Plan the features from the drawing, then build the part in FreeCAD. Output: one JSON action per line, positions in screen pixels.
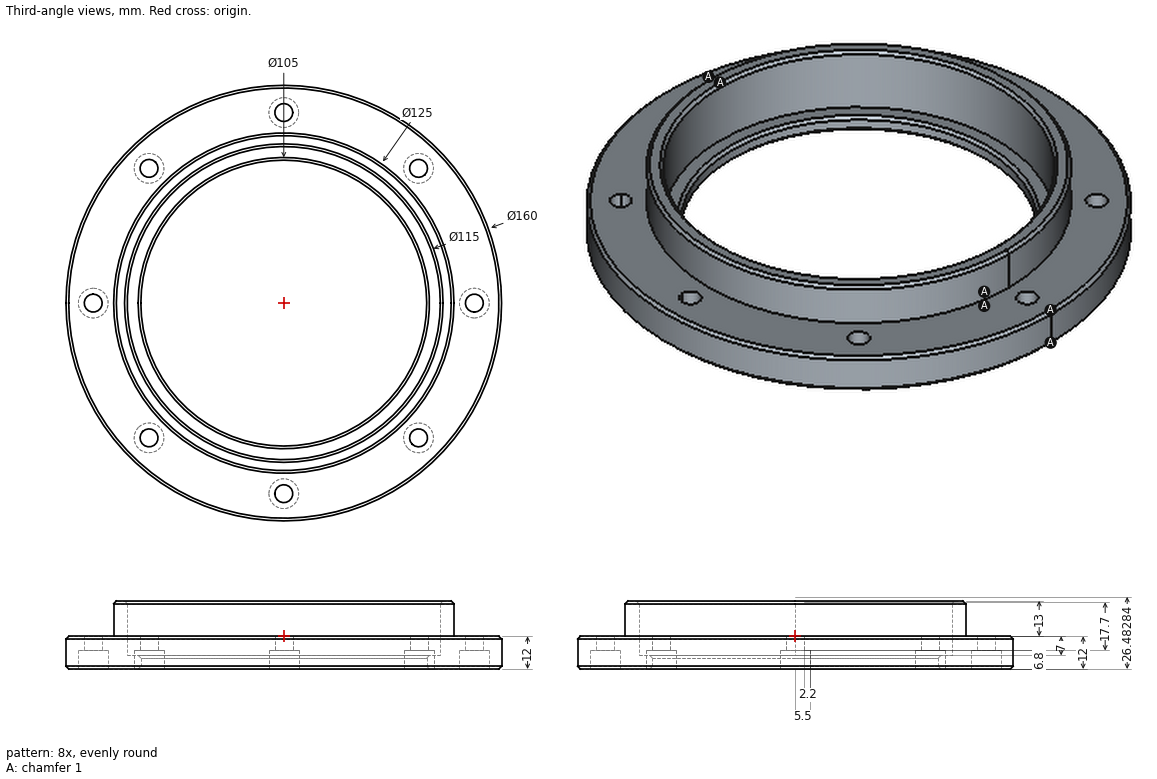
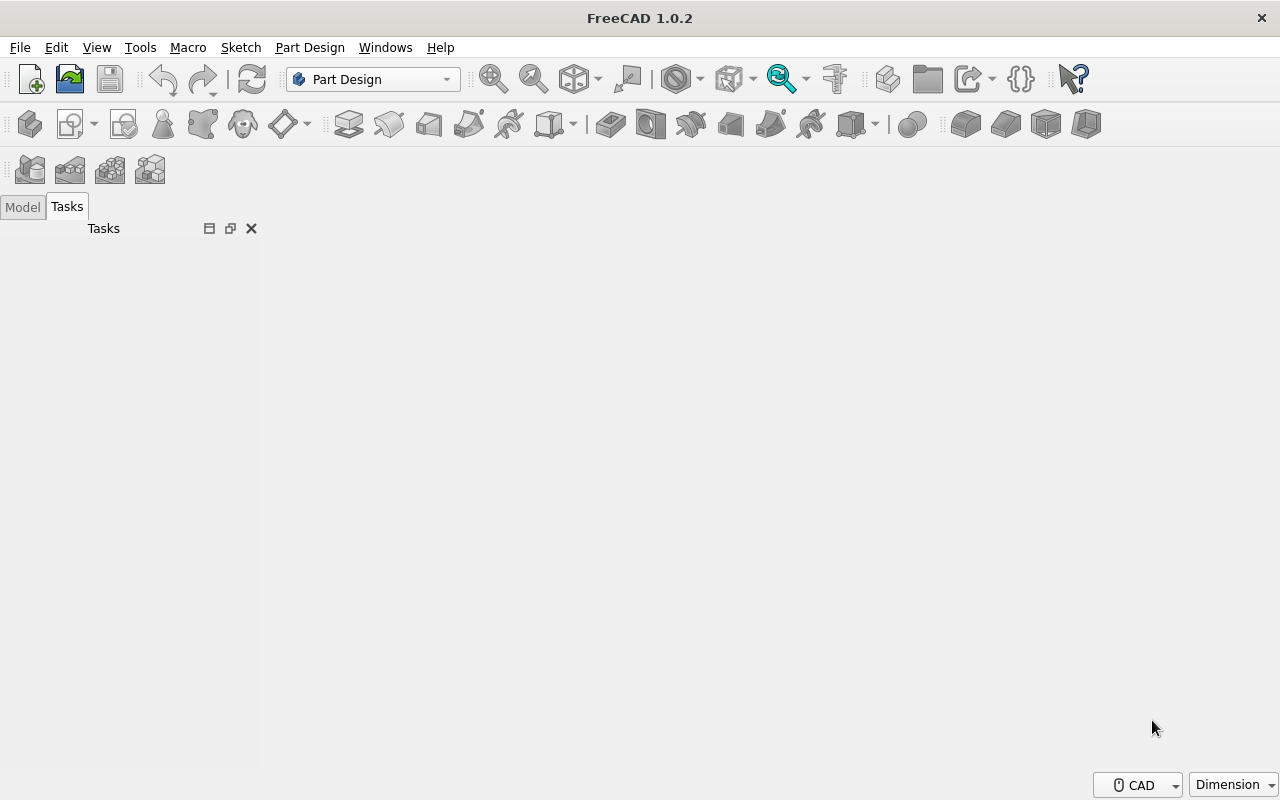
{"action": "key", "text": "ctrl+n"}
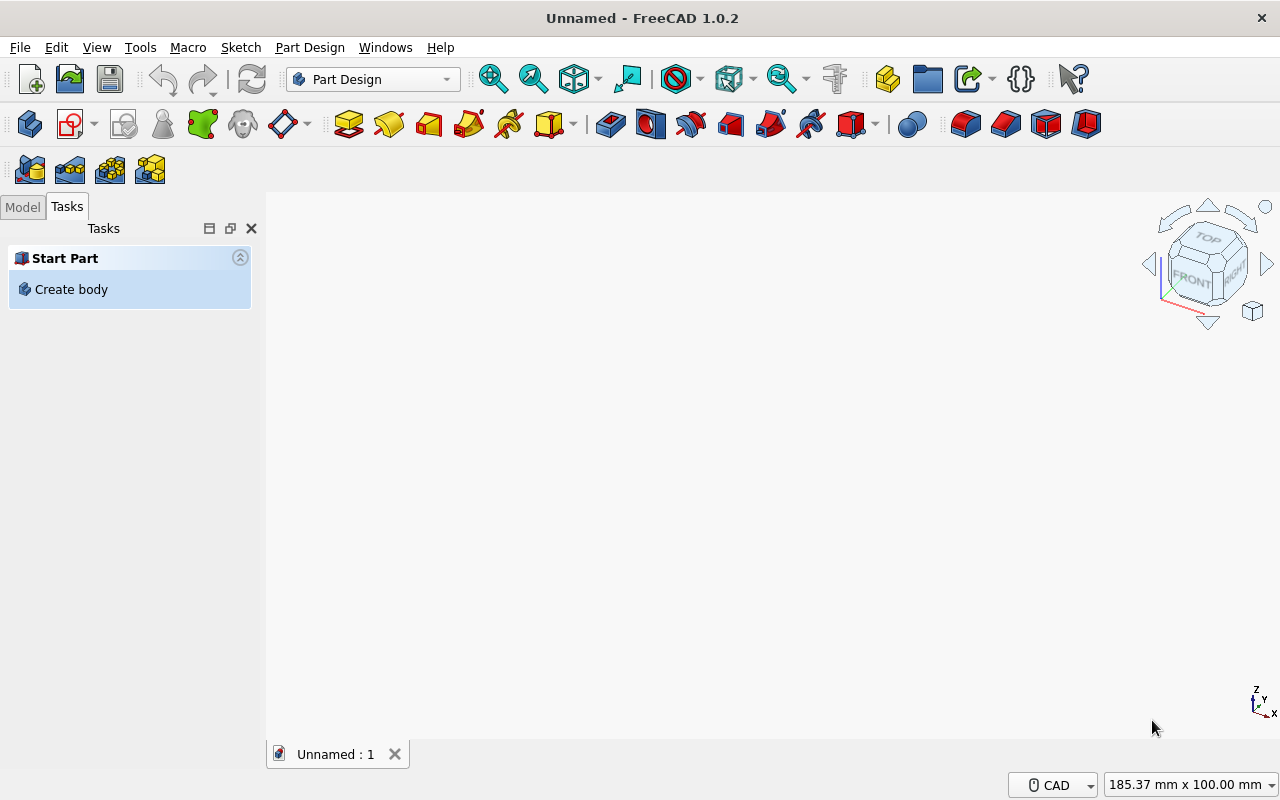
{"action": "left_click", "coordinate": [70, 124]}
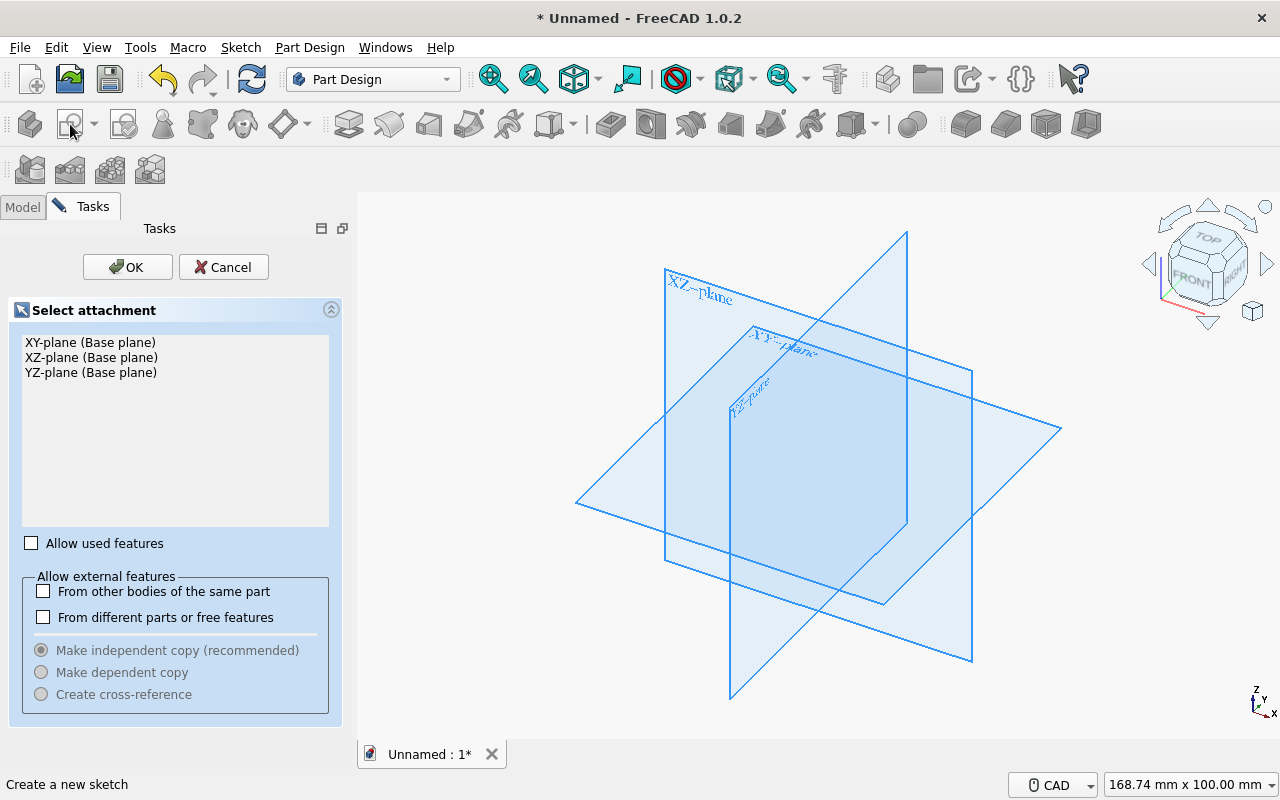
{"action": "left_click", "coordinate": [82, 342]}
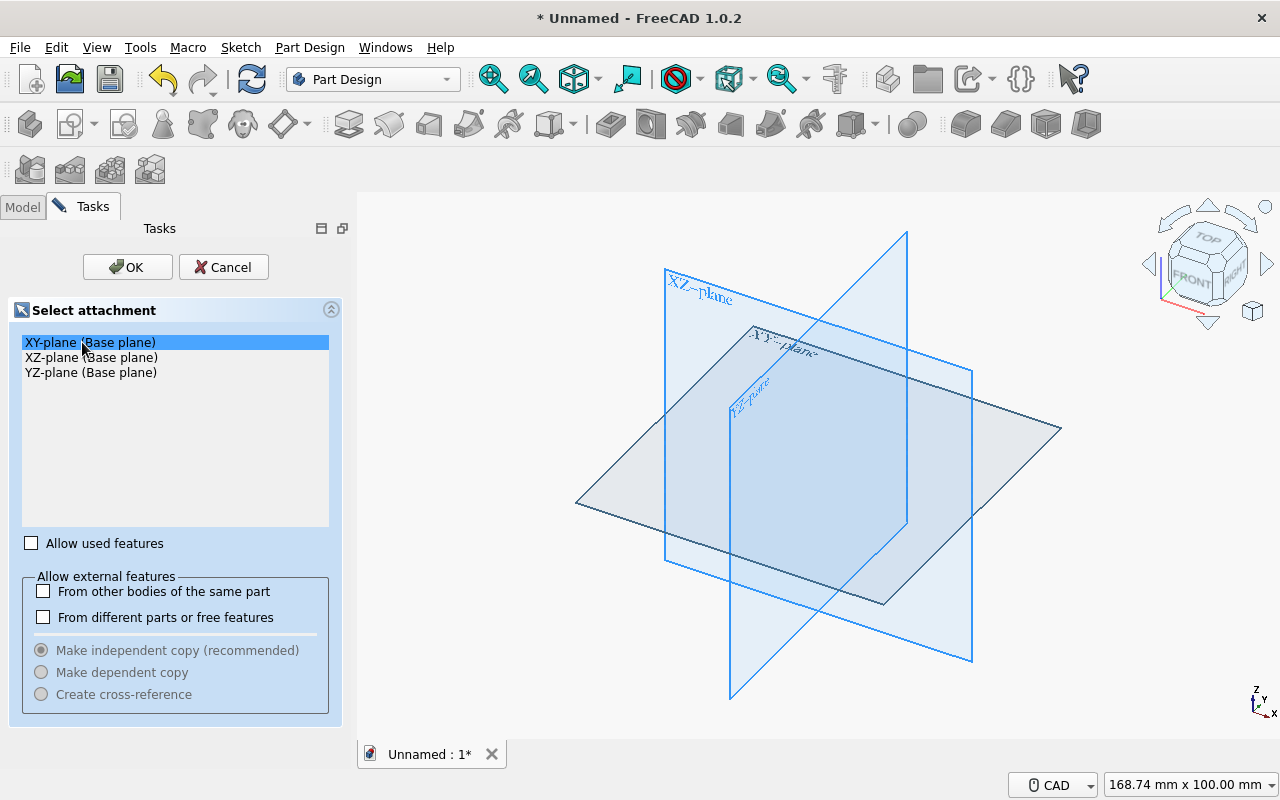
{"action": "left_click", "coordinate": [128, 267]}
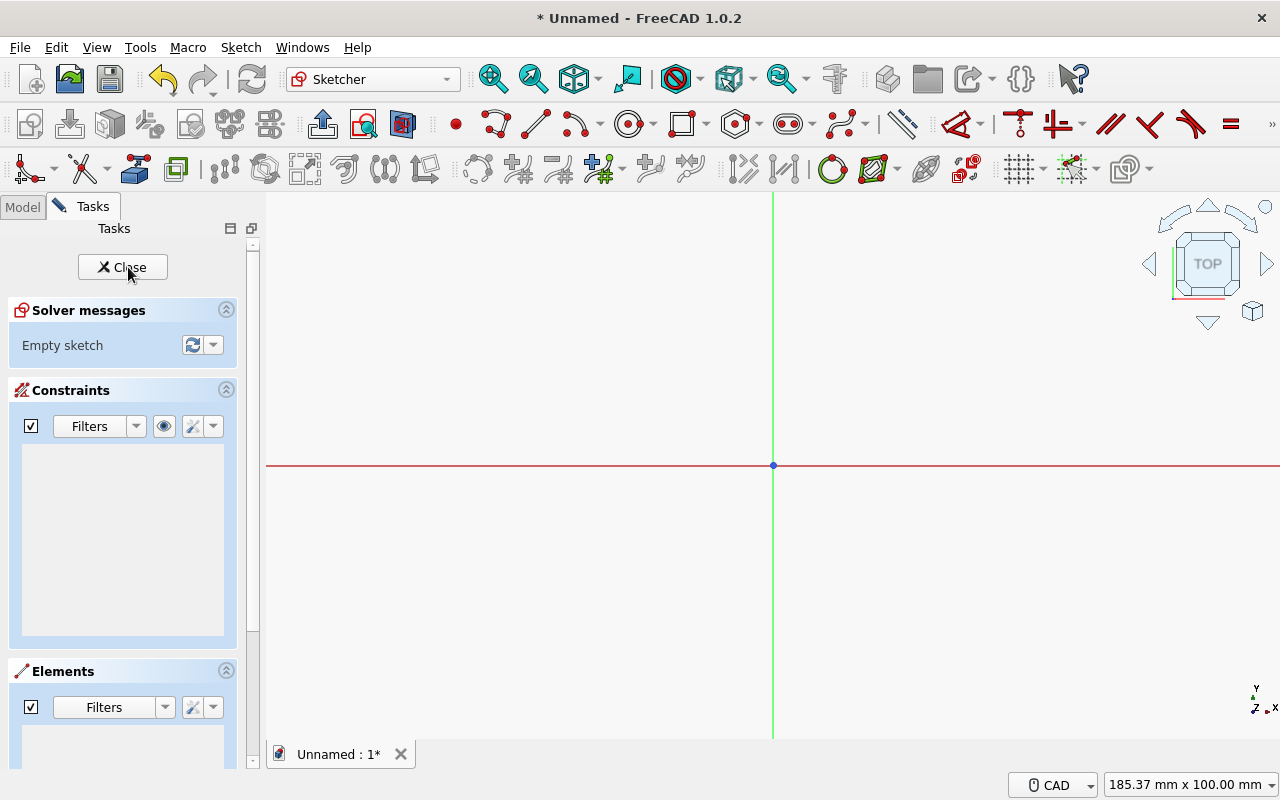
{"action": "scroll", "coordinate": [621, 466], "scroll_direction": "down", "scroll_amount": 3}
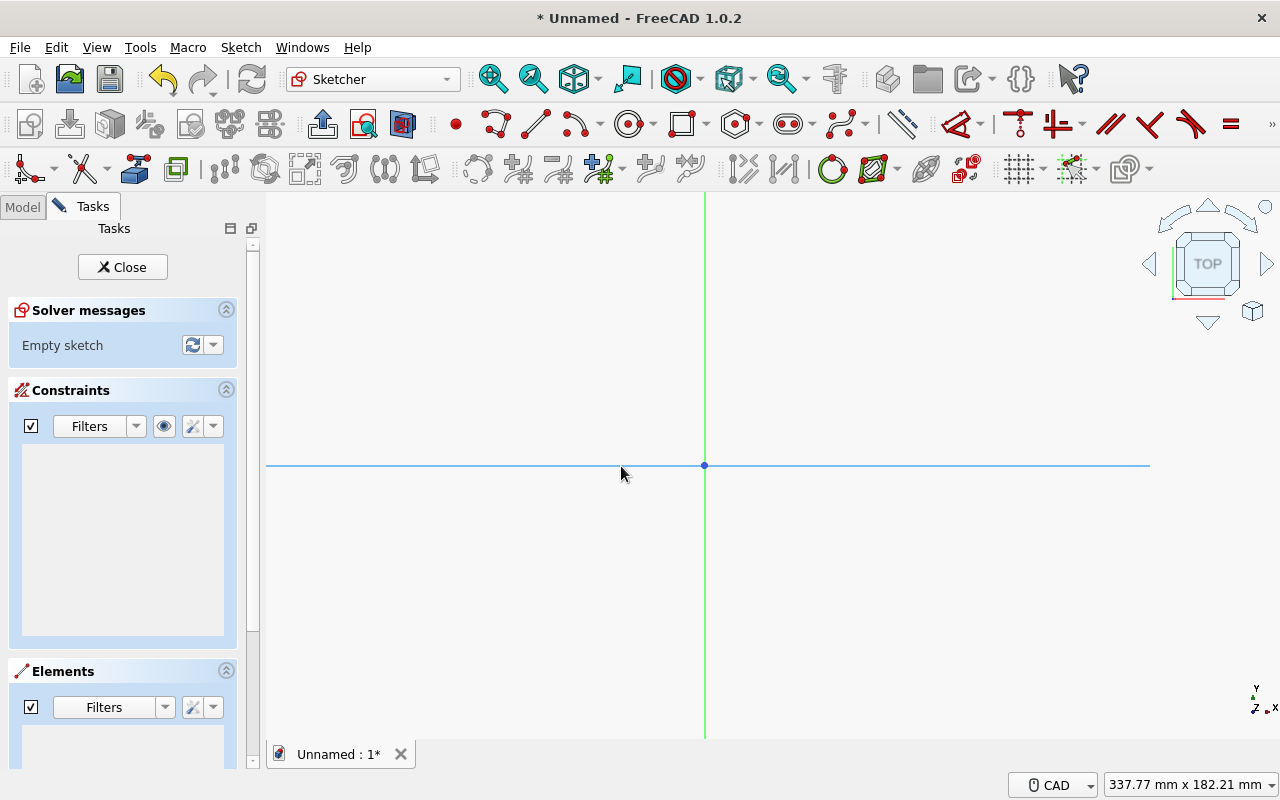
{"action": "left_click", "coordinate": [630, 124]}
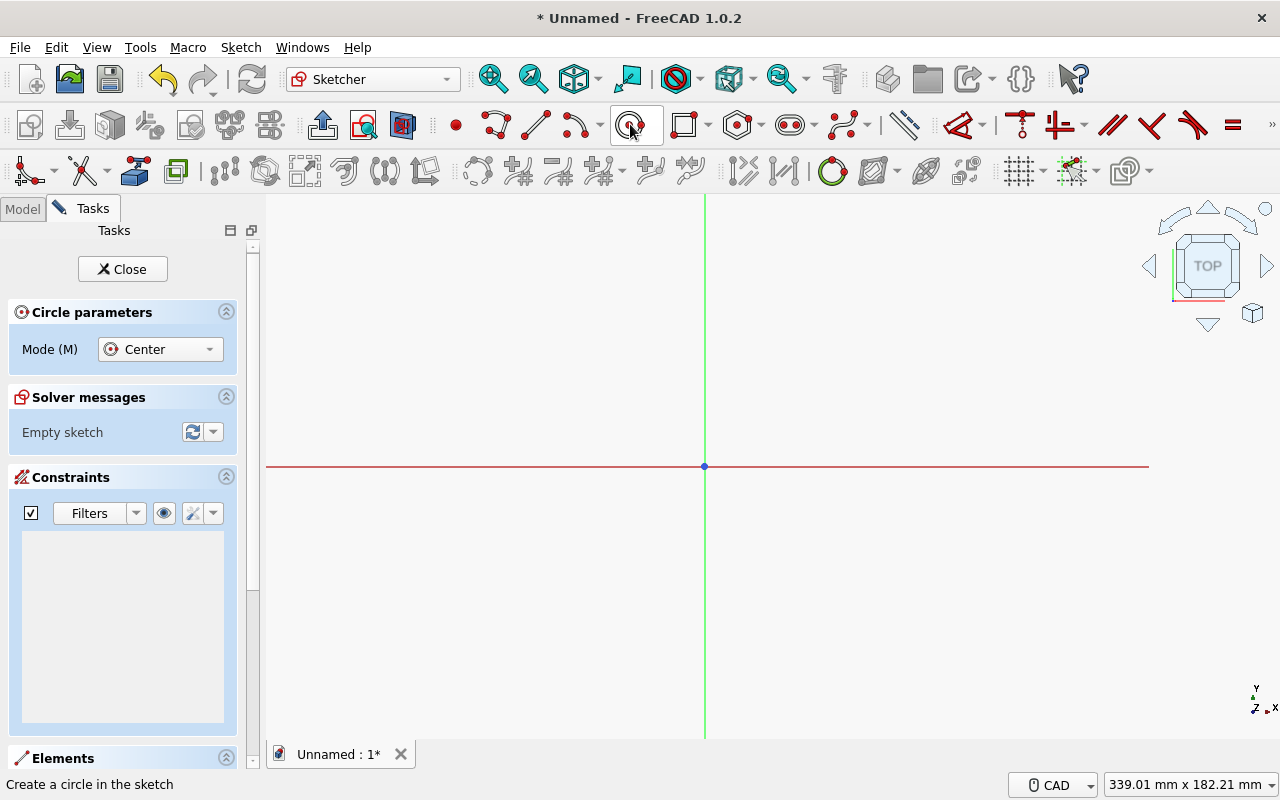
{"action": "left_click", "coordinate": [705, 467]}
{"action": "left_click", "coordinate": [837, 335]}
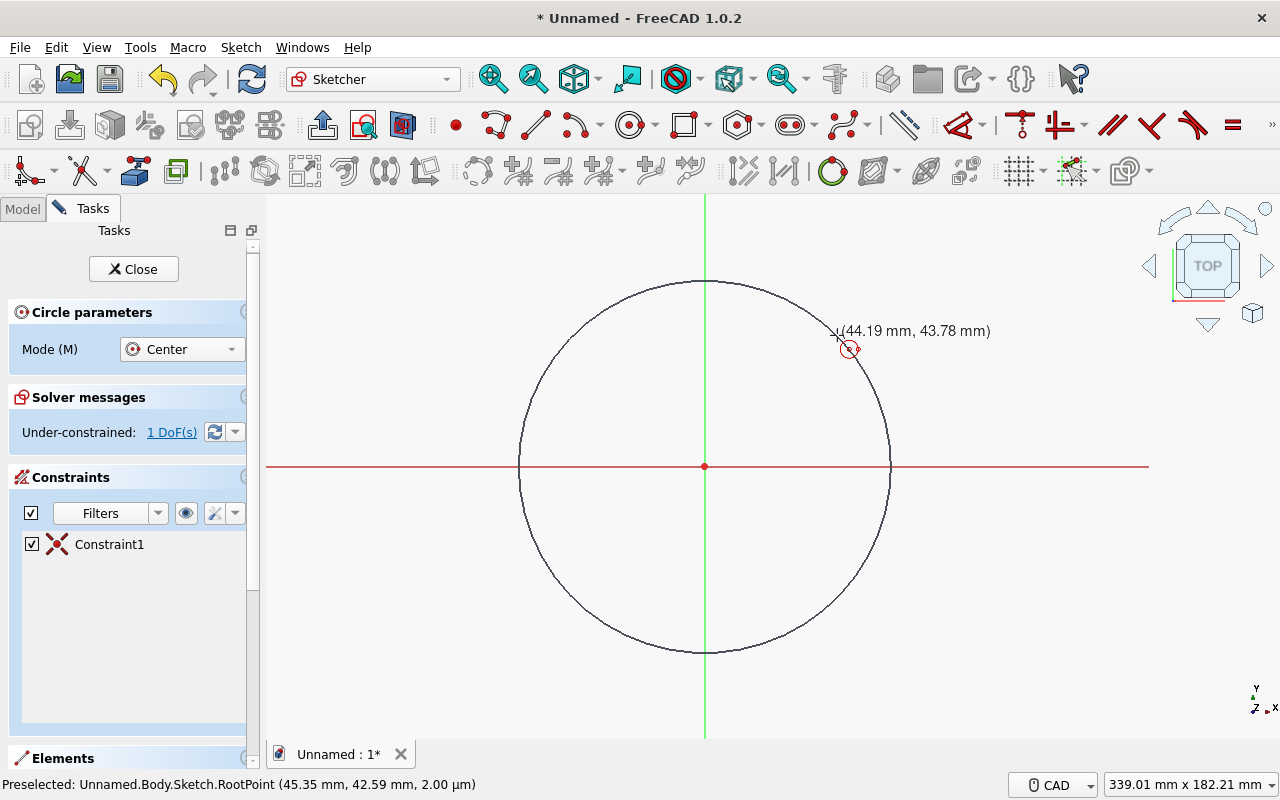
{"action": "left_click", "coordinate": [705, 467]}
{"action": "left_click", "coordinate": [826, 345]}
{"action": "key", "text": "Escape"}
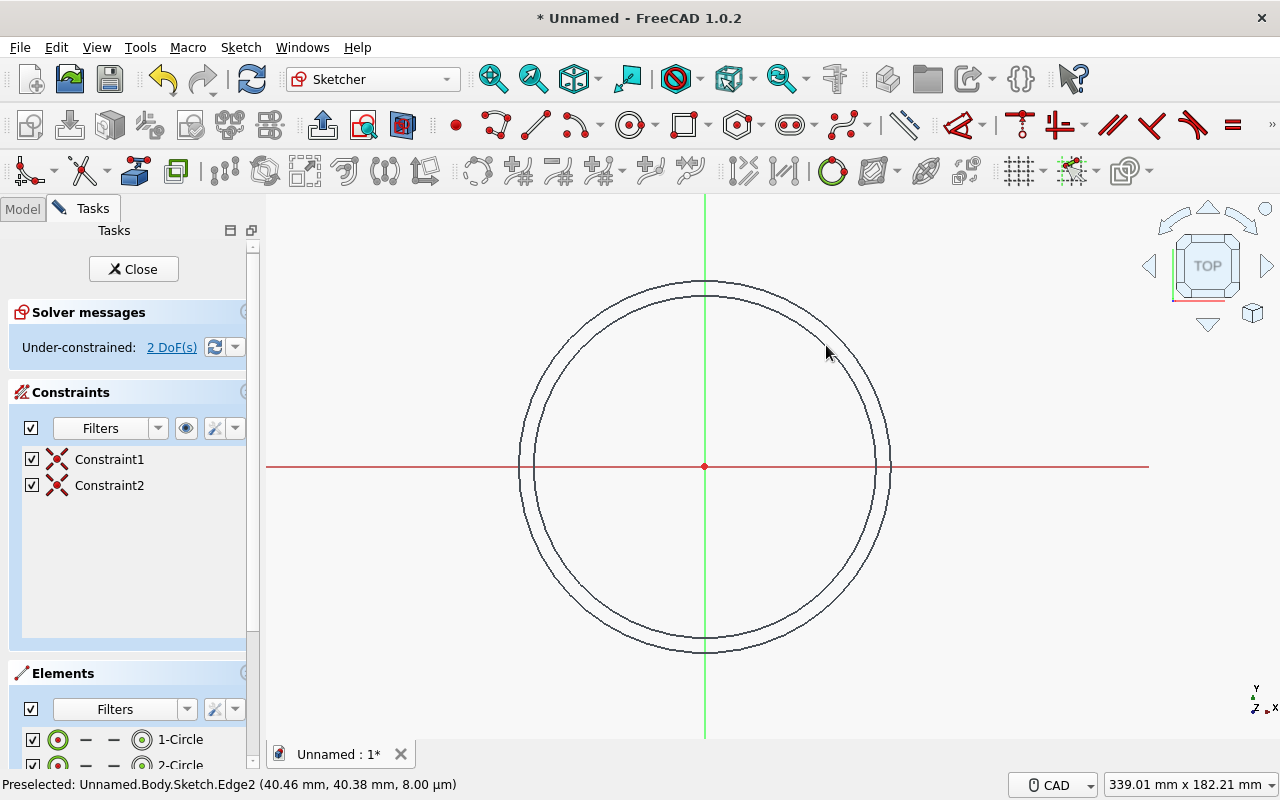
{"action": "left_click", "coordinate": [836, 335]}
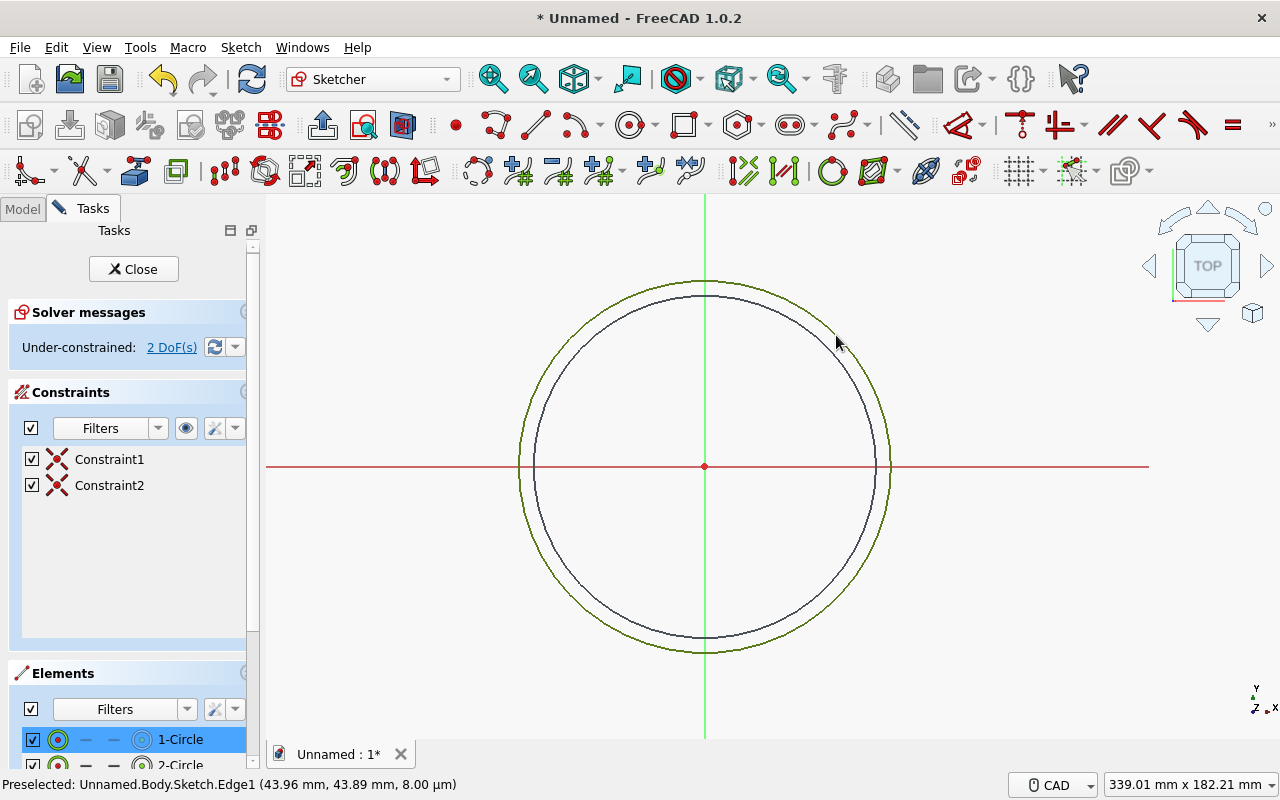
{"action": "key", "text": "k o"}